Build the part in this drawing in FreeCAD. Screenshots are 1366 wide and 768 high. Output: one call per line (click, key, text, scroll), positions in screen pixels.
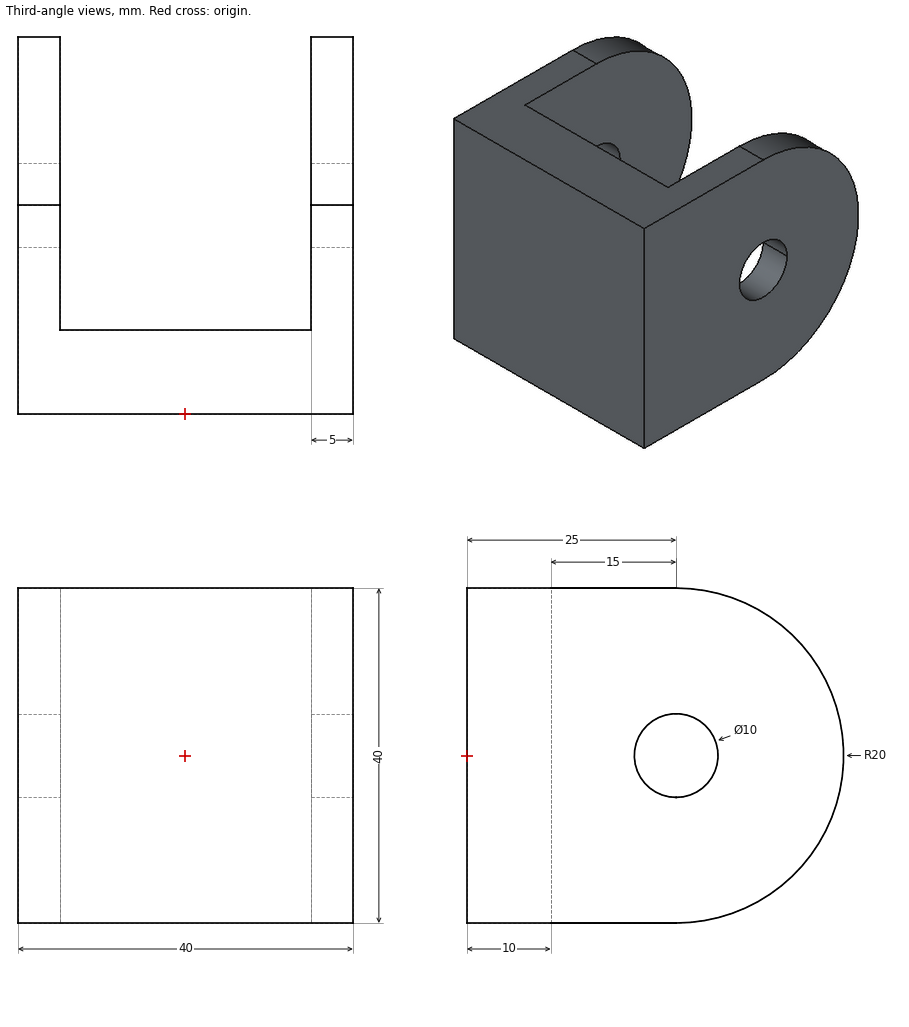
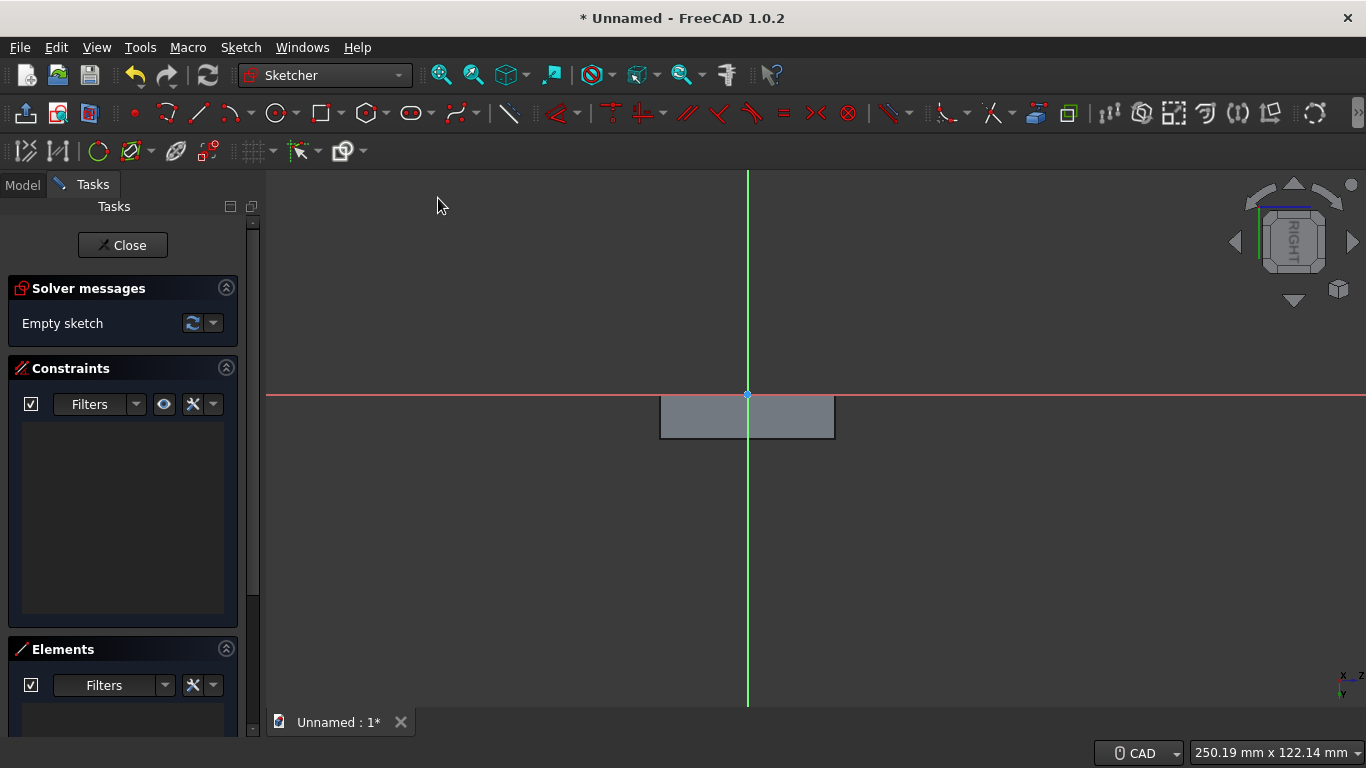
scroll(748, 561, up, 3)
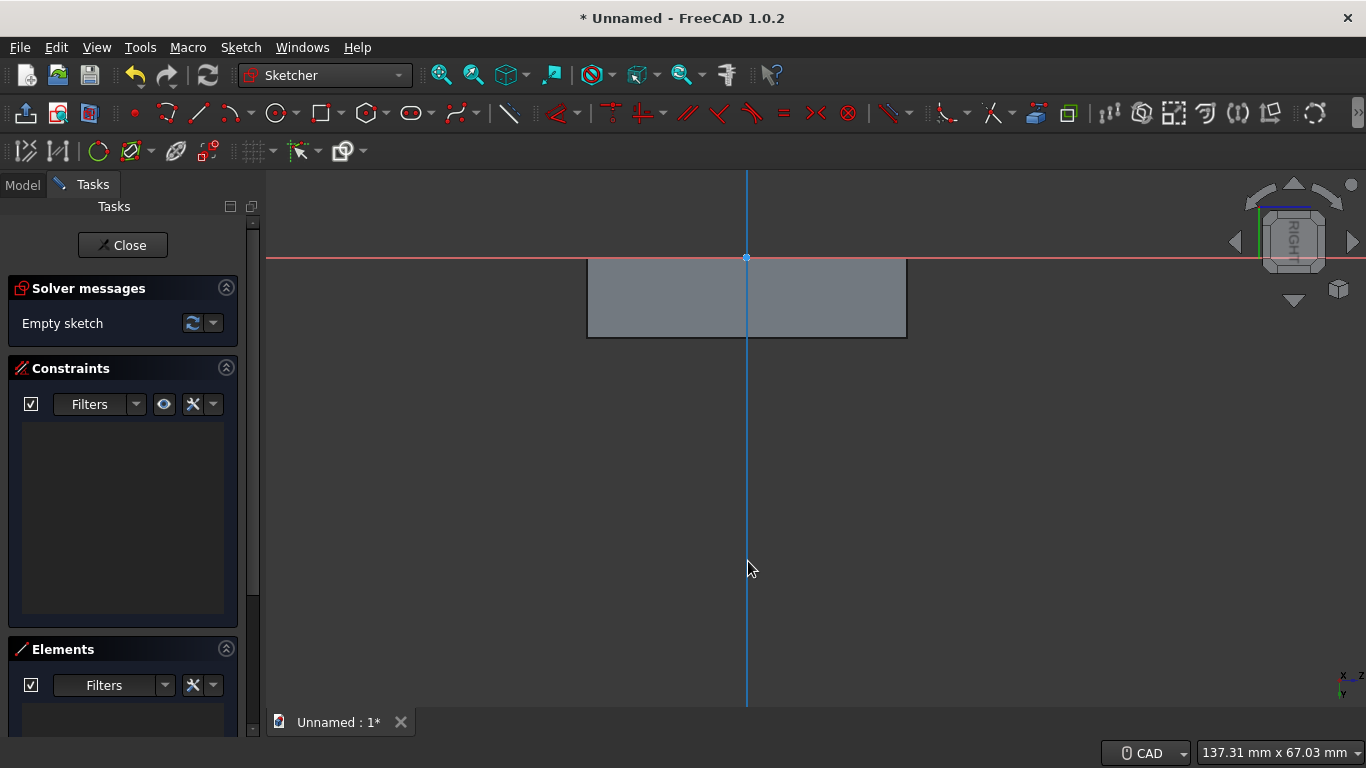
click(168, 114)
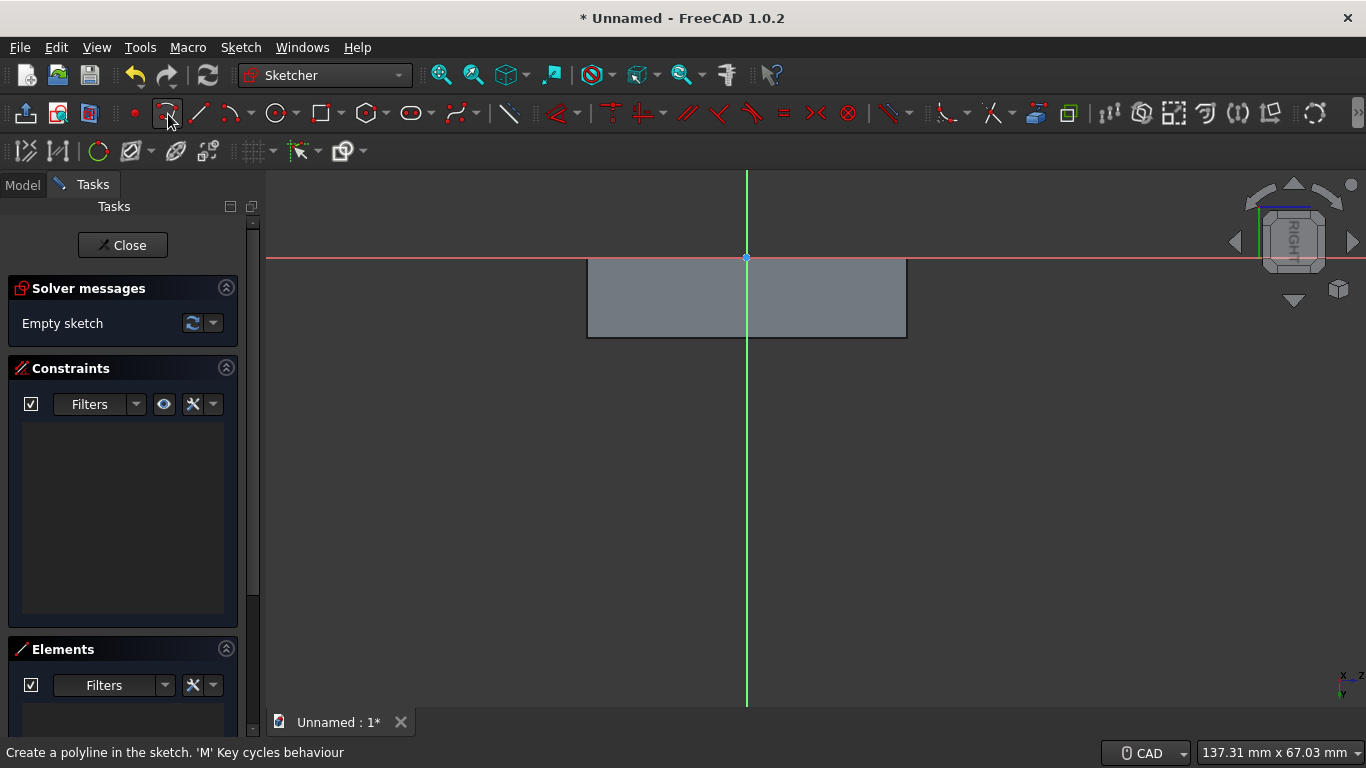
click(907, 458)
click(907, 338)
click(587, 338)
click(587, 458)
right_click(587, 458)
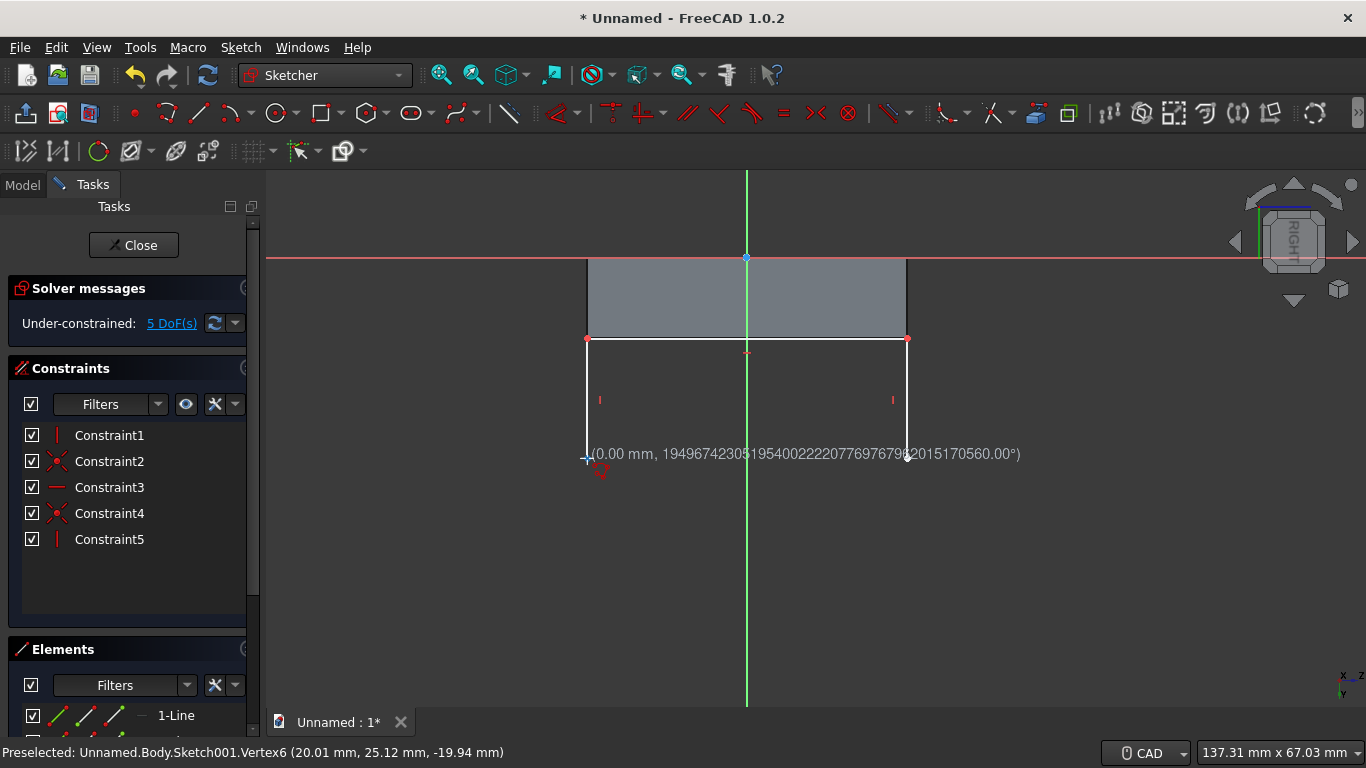
click(254, 114)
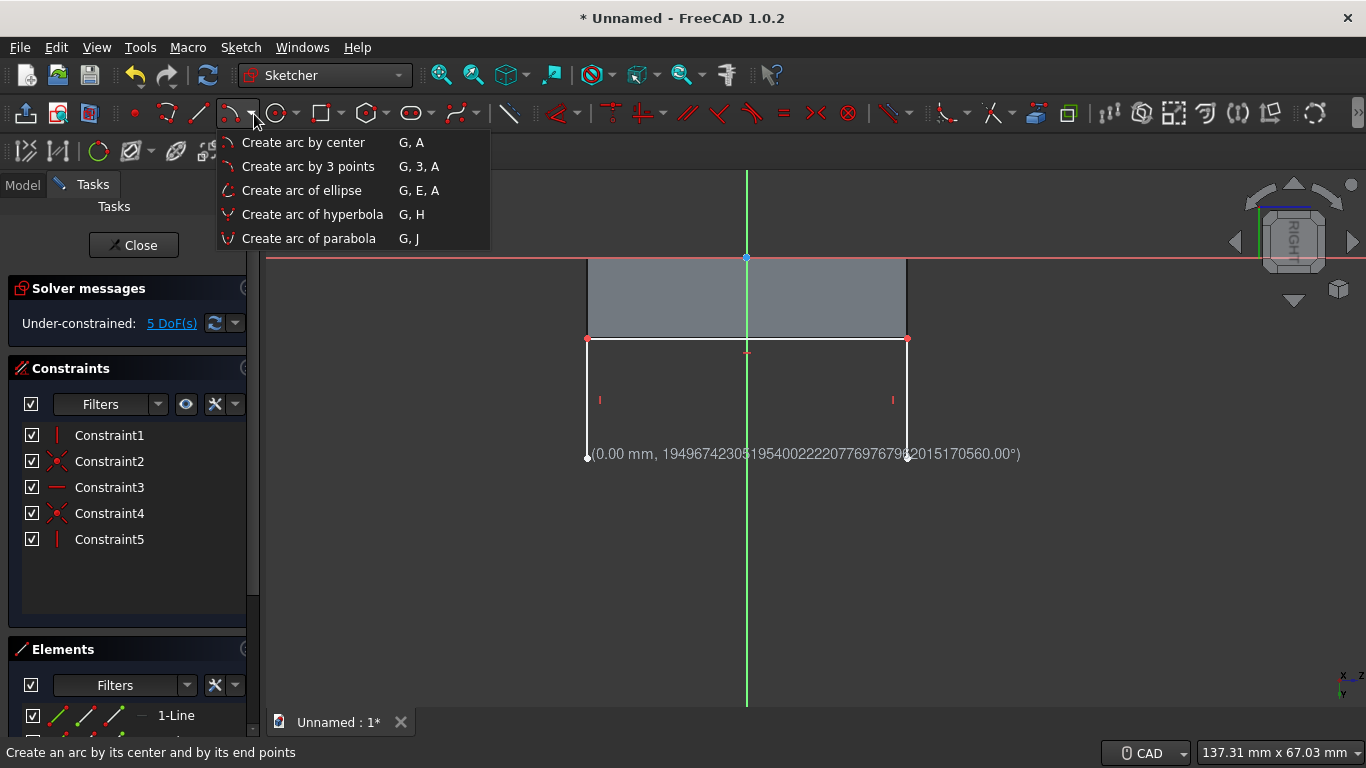
click(354, 166)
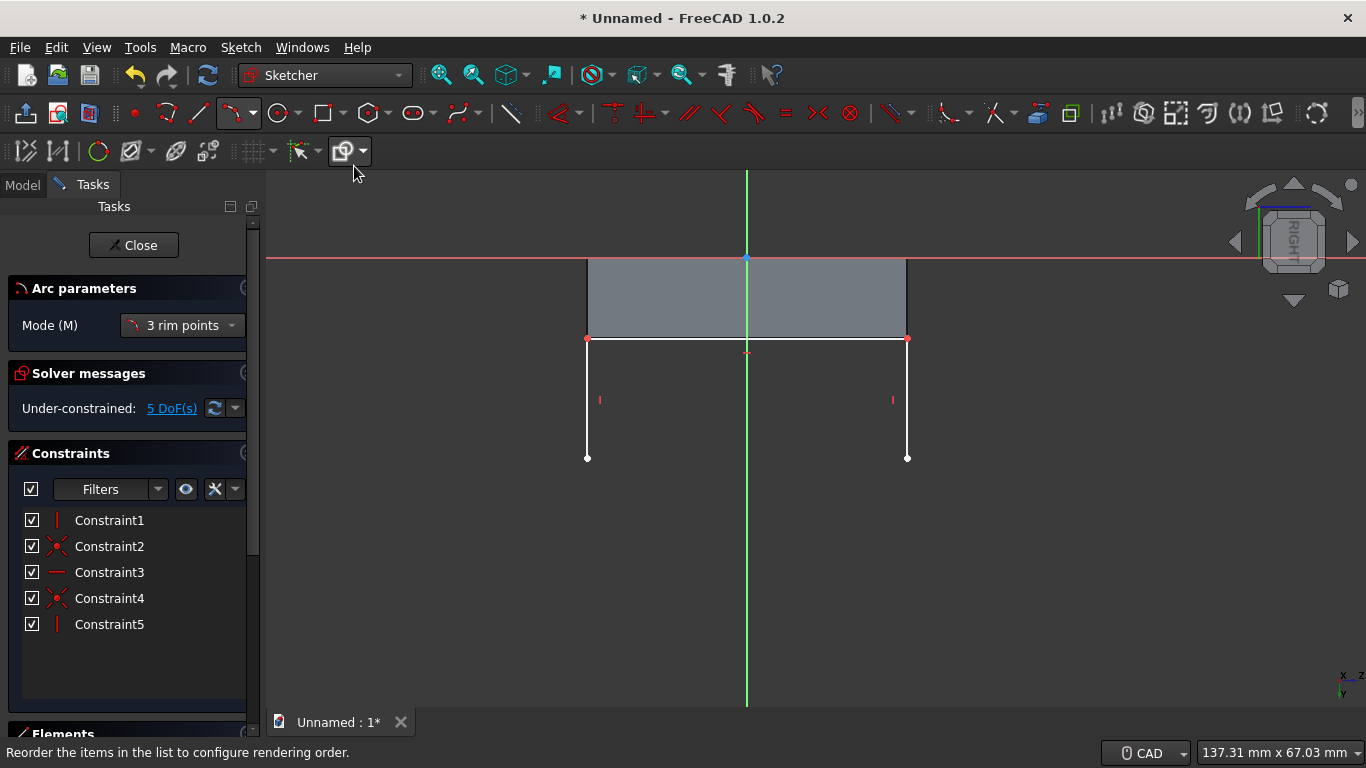
click(587, 459)
click(907, 459)
click(697, 610)
key(Escape)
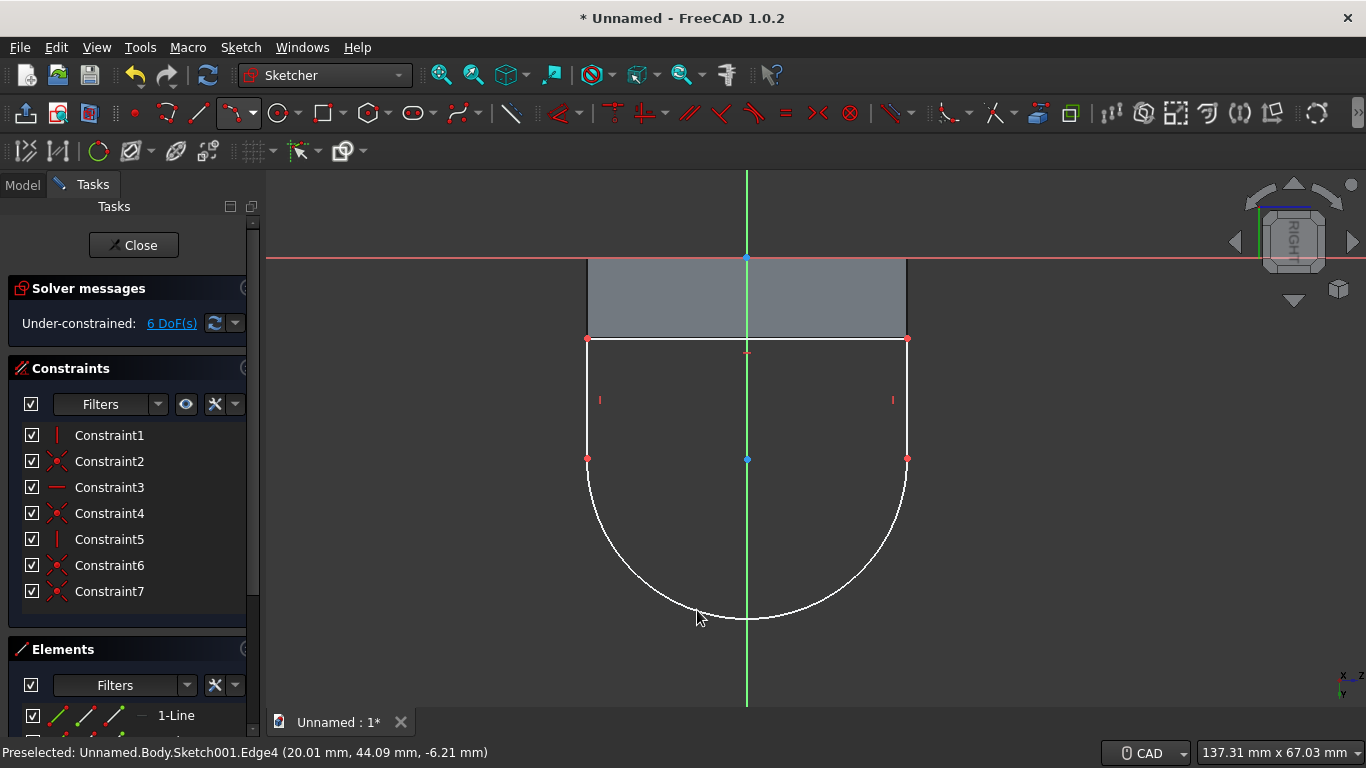
click(907, 423)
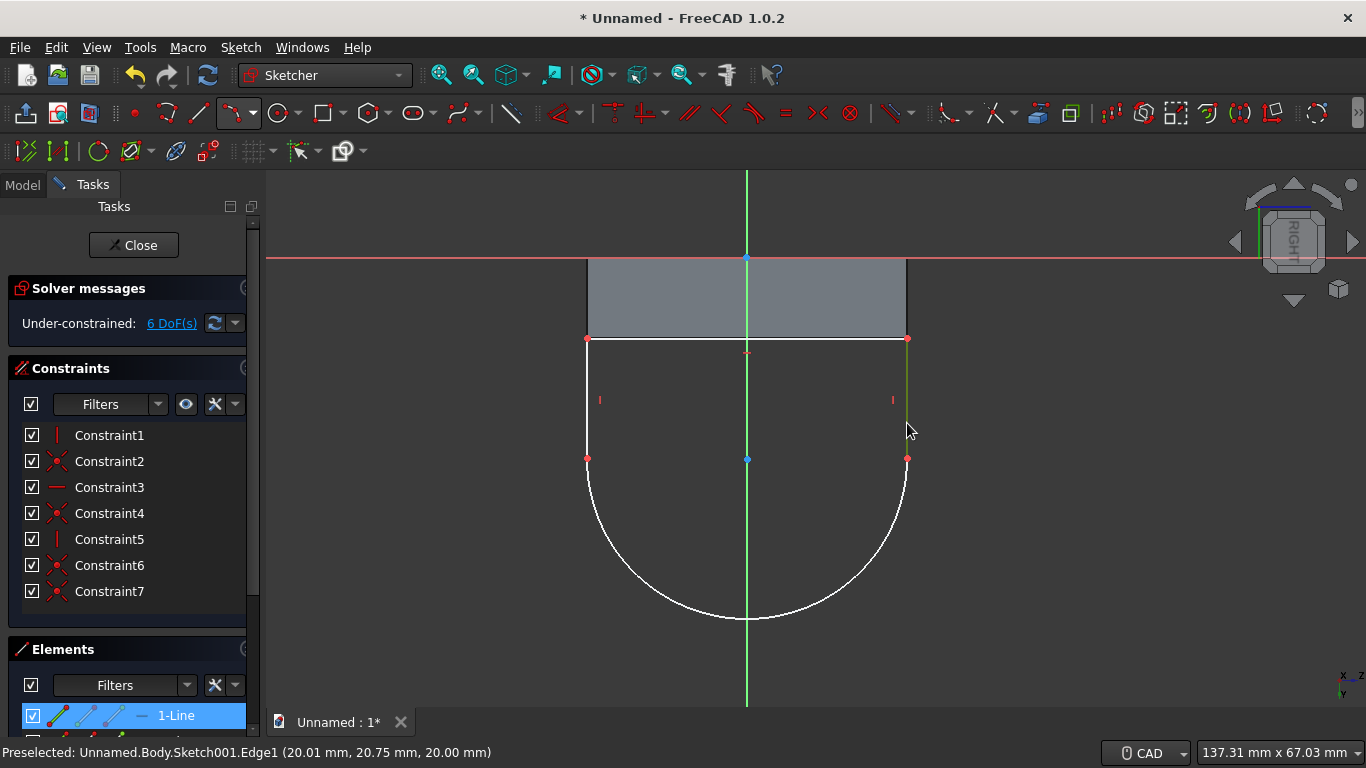
click(653, 588)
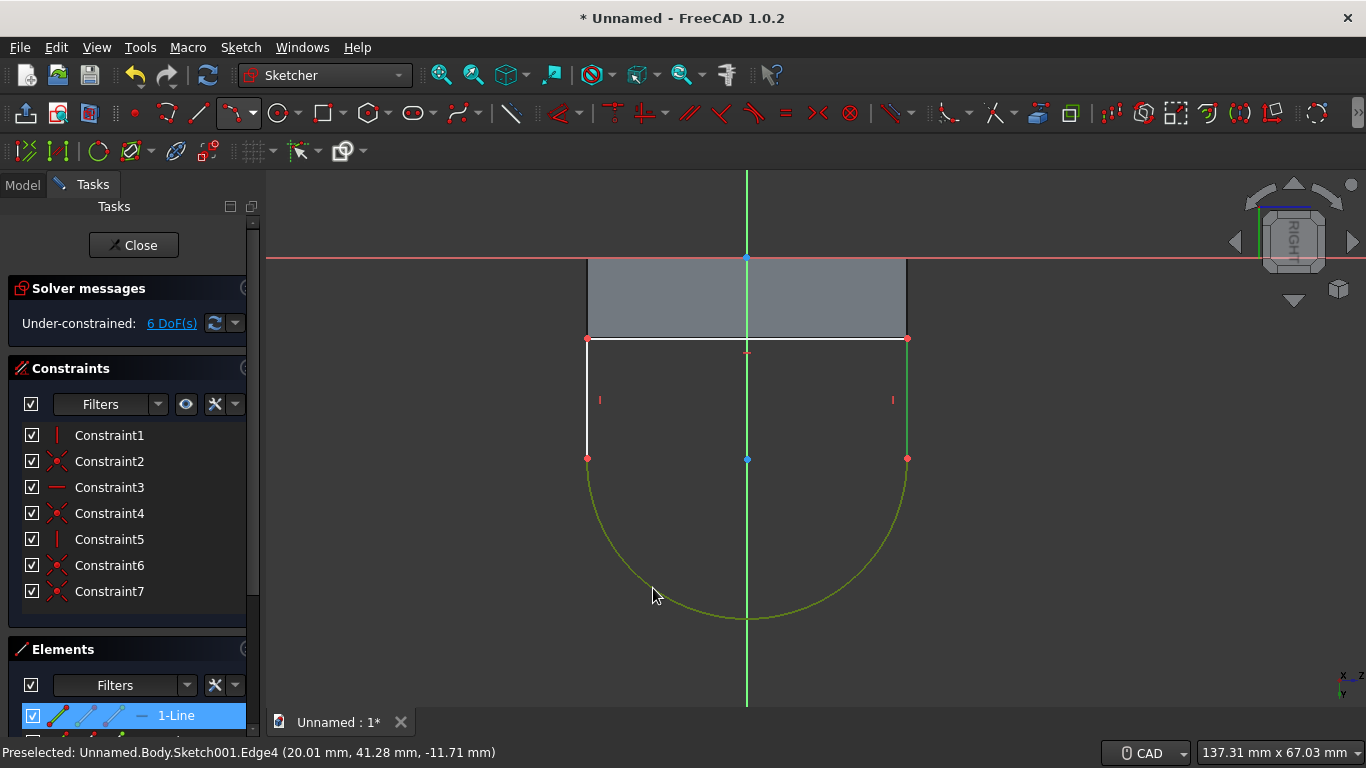
click(754, 114)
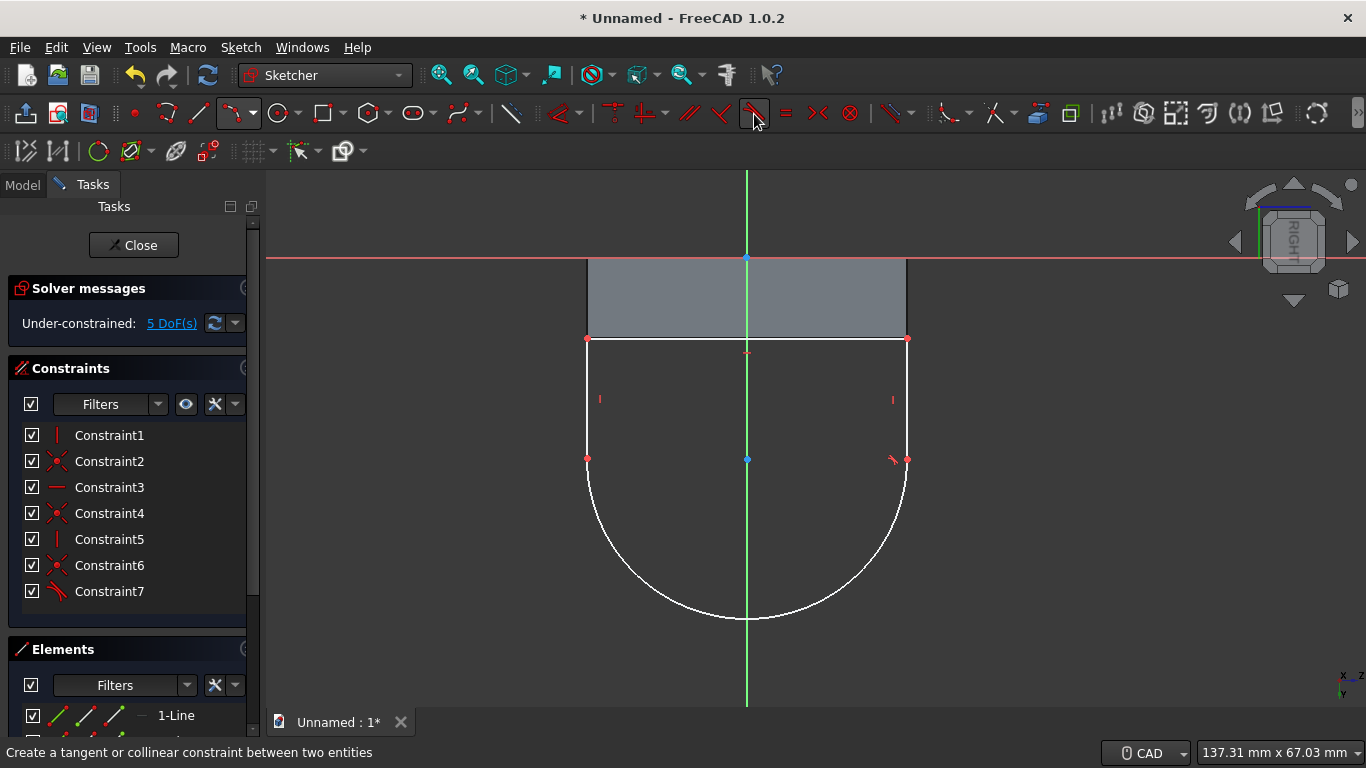
click(587, 375)